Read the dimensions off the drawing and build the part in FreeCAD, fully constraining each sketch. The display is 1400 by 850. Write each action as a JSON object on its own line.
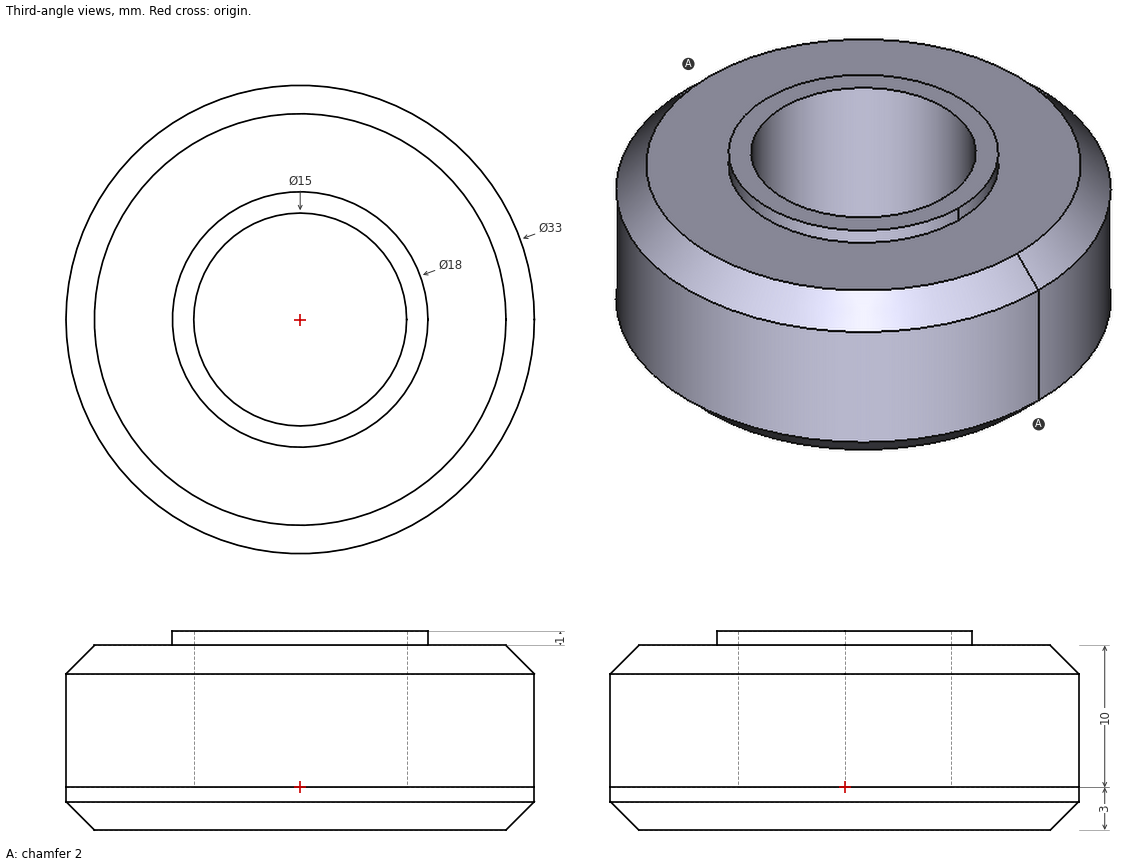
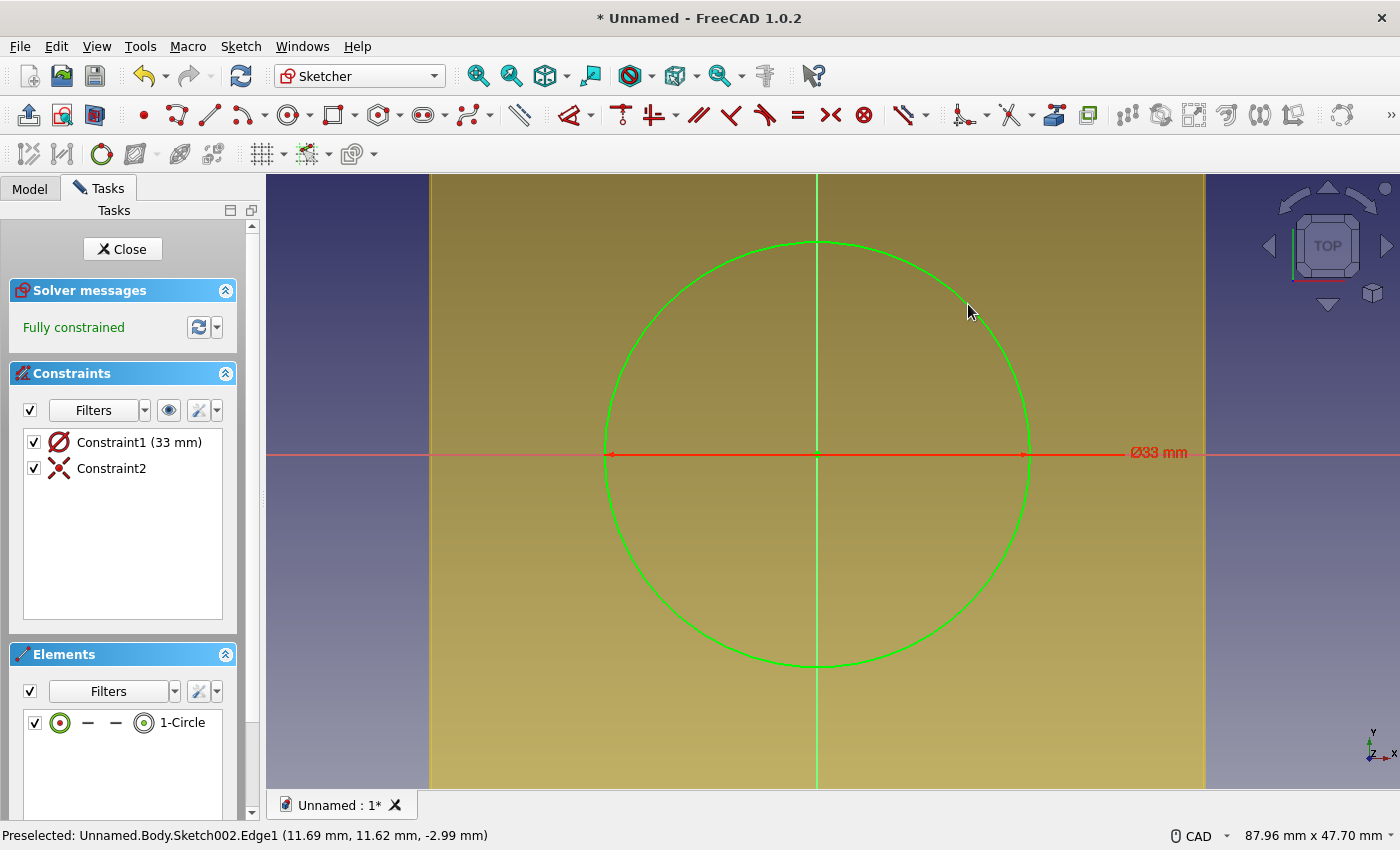
{"action": "left_click", "coordinate": [123, 249]}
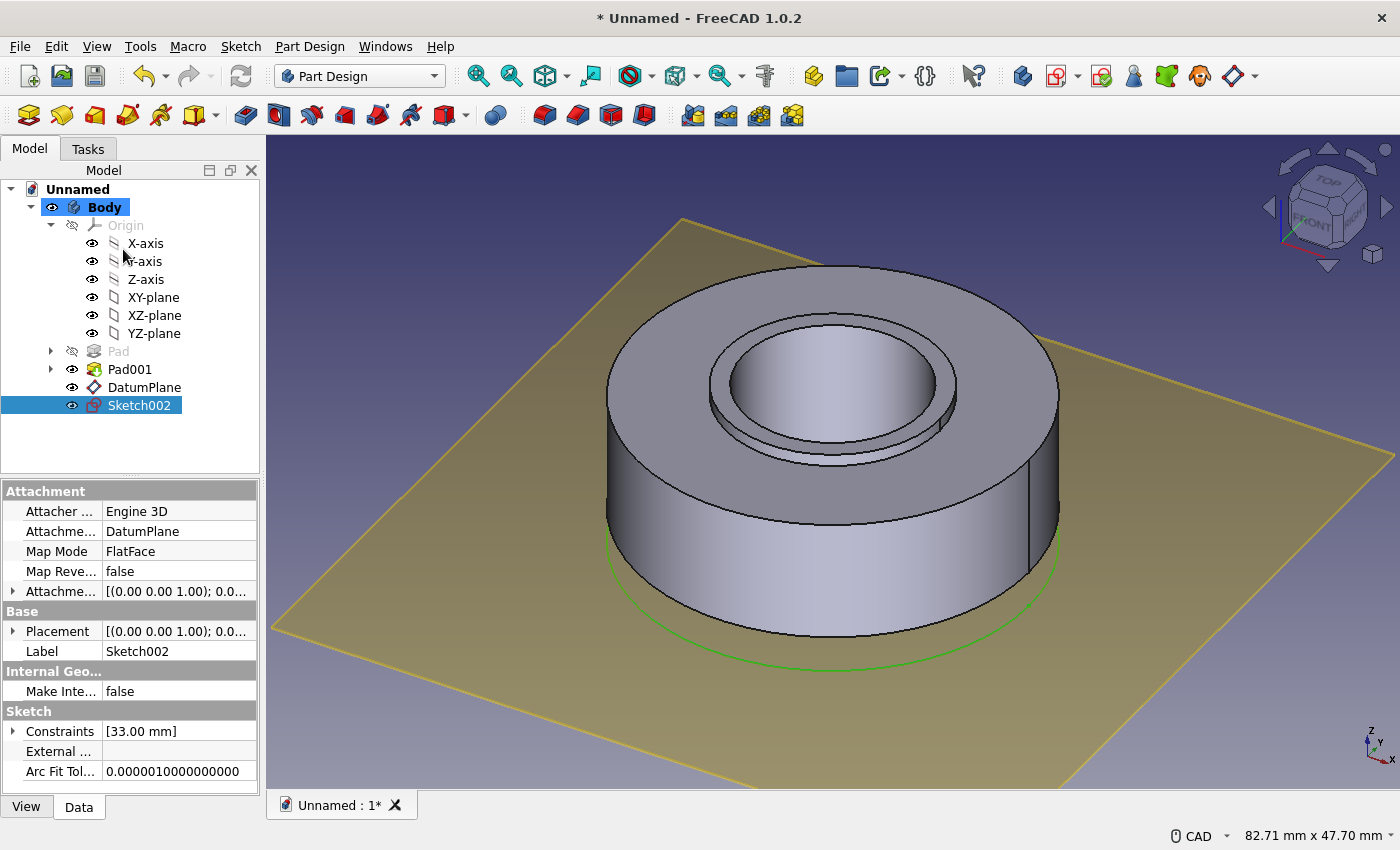
{"action": "left_click", "coordinate": [29, 116]}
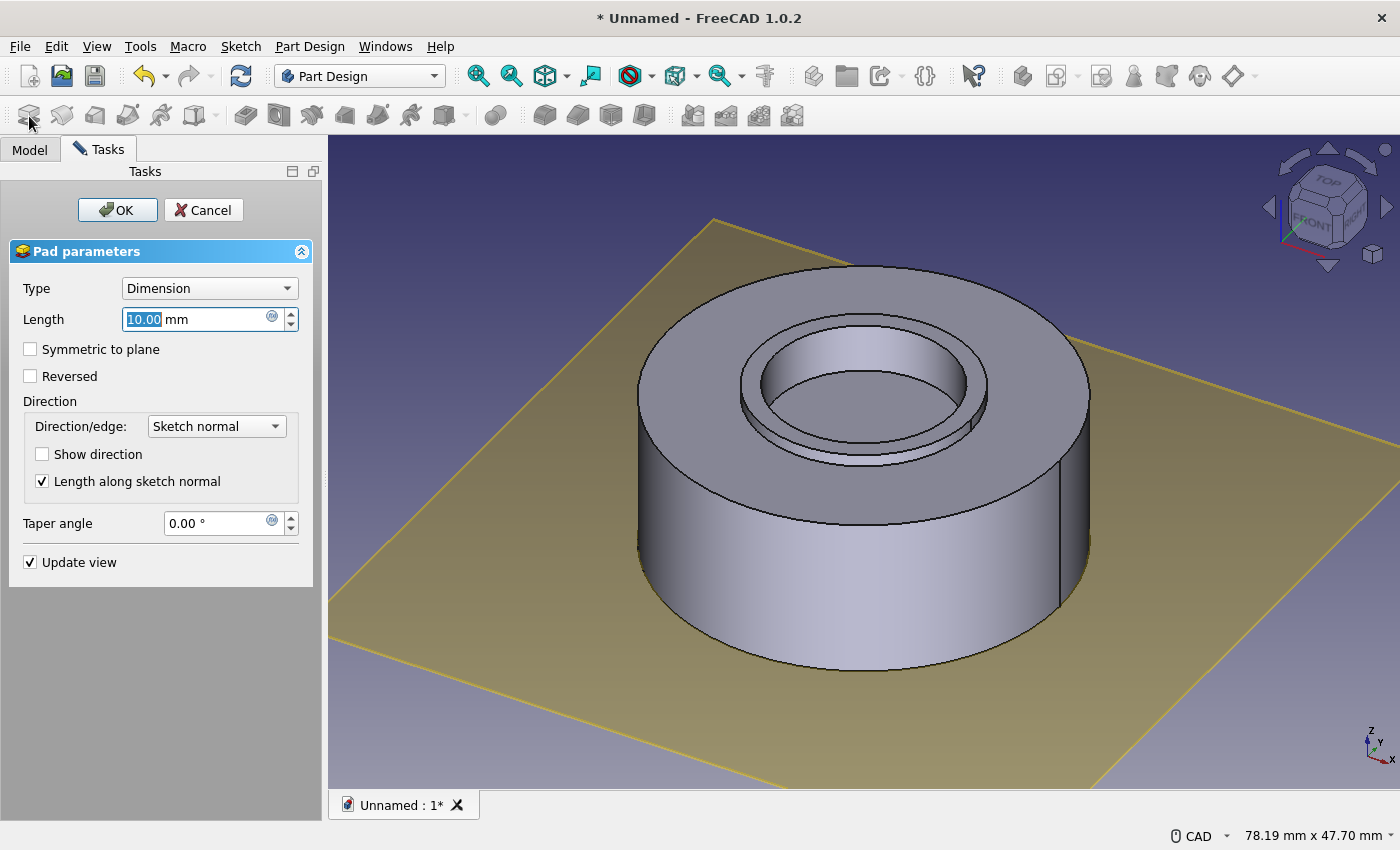
{"action": "type", "text": "3"}
{"action": "key", "text": "Tab"}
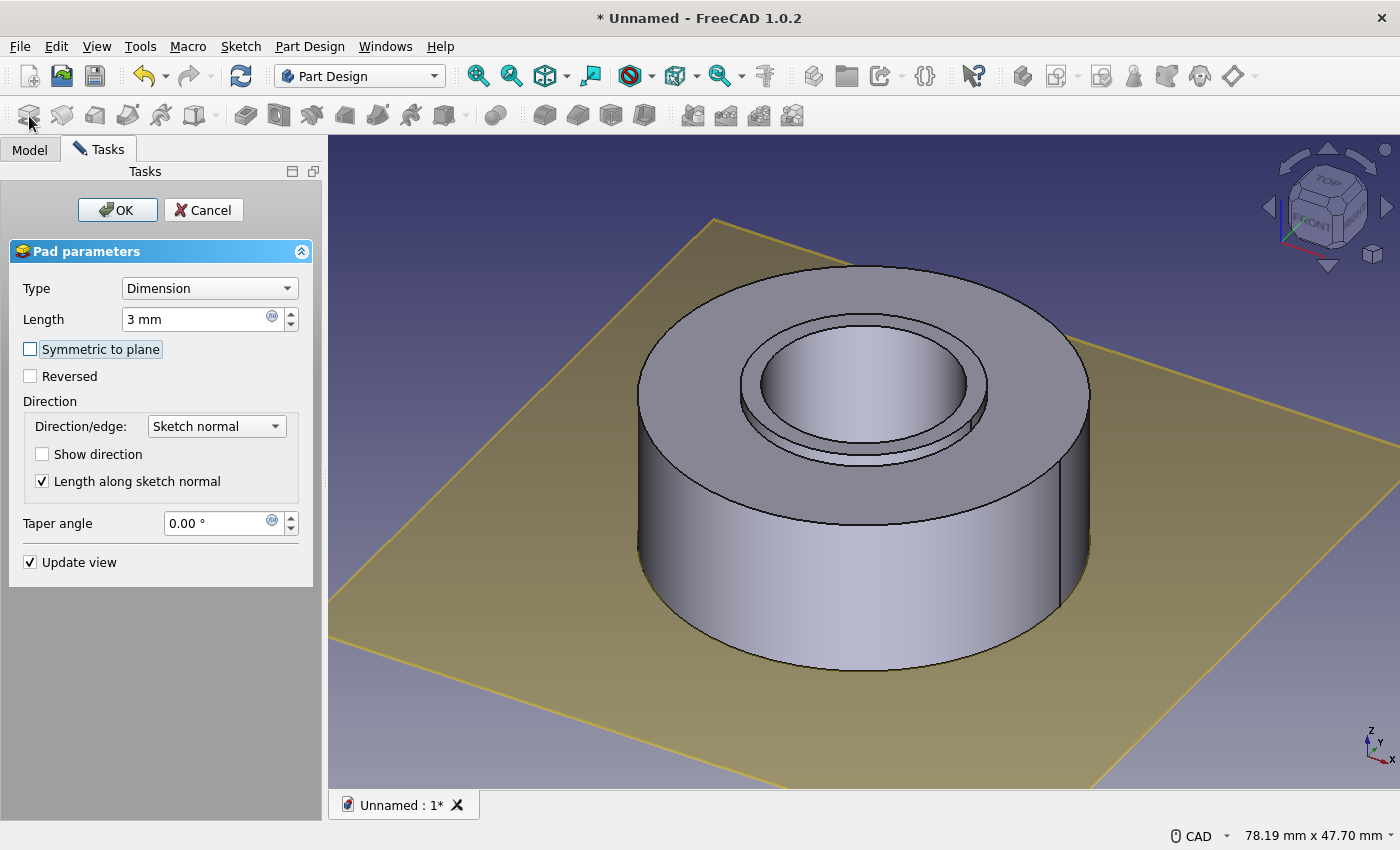
{"action": "left_click", "coordinate": [118, 210]}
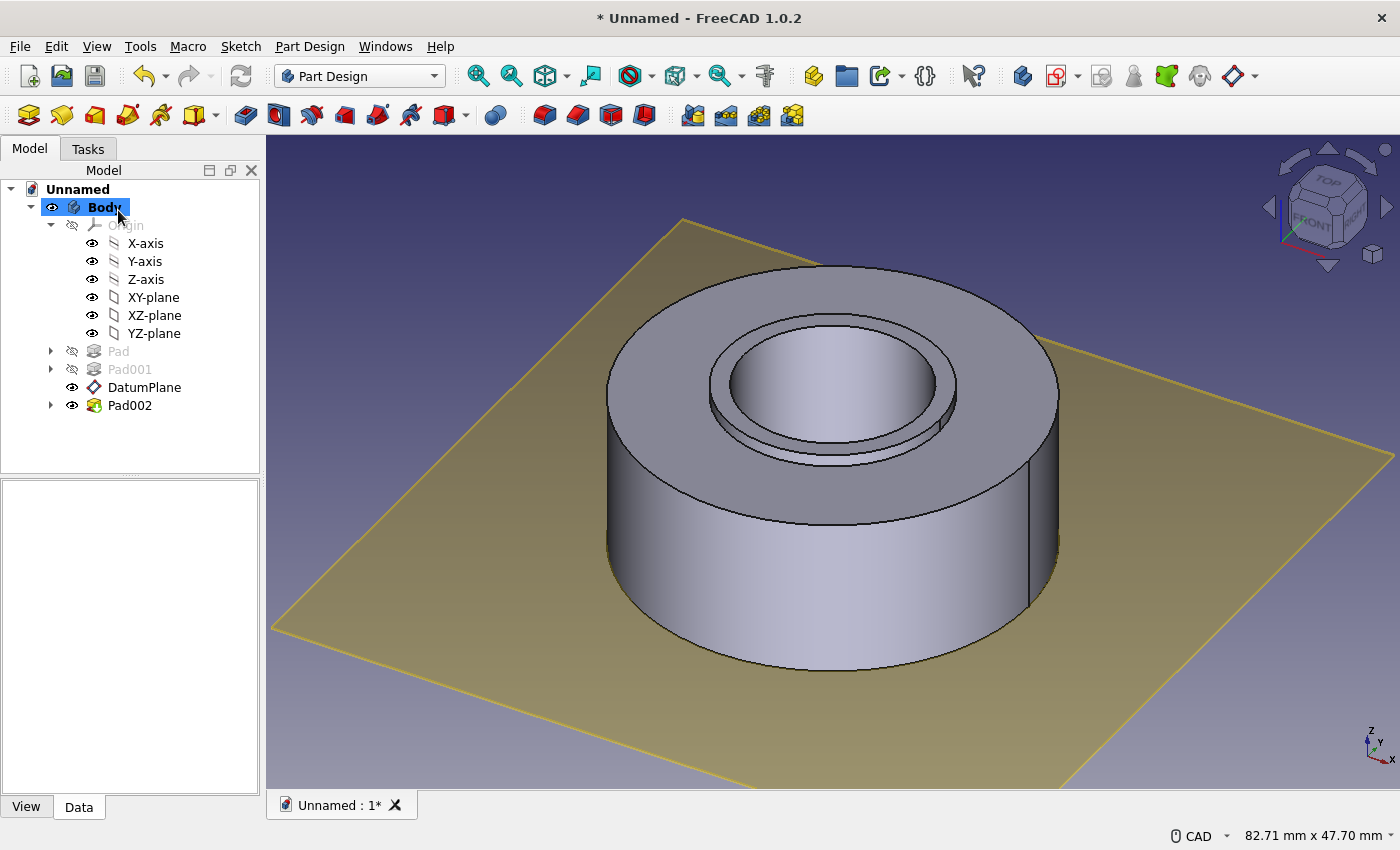
{"action": "left_click", "coordinate": [117, 387]}
{"action": "key", "text": "space"}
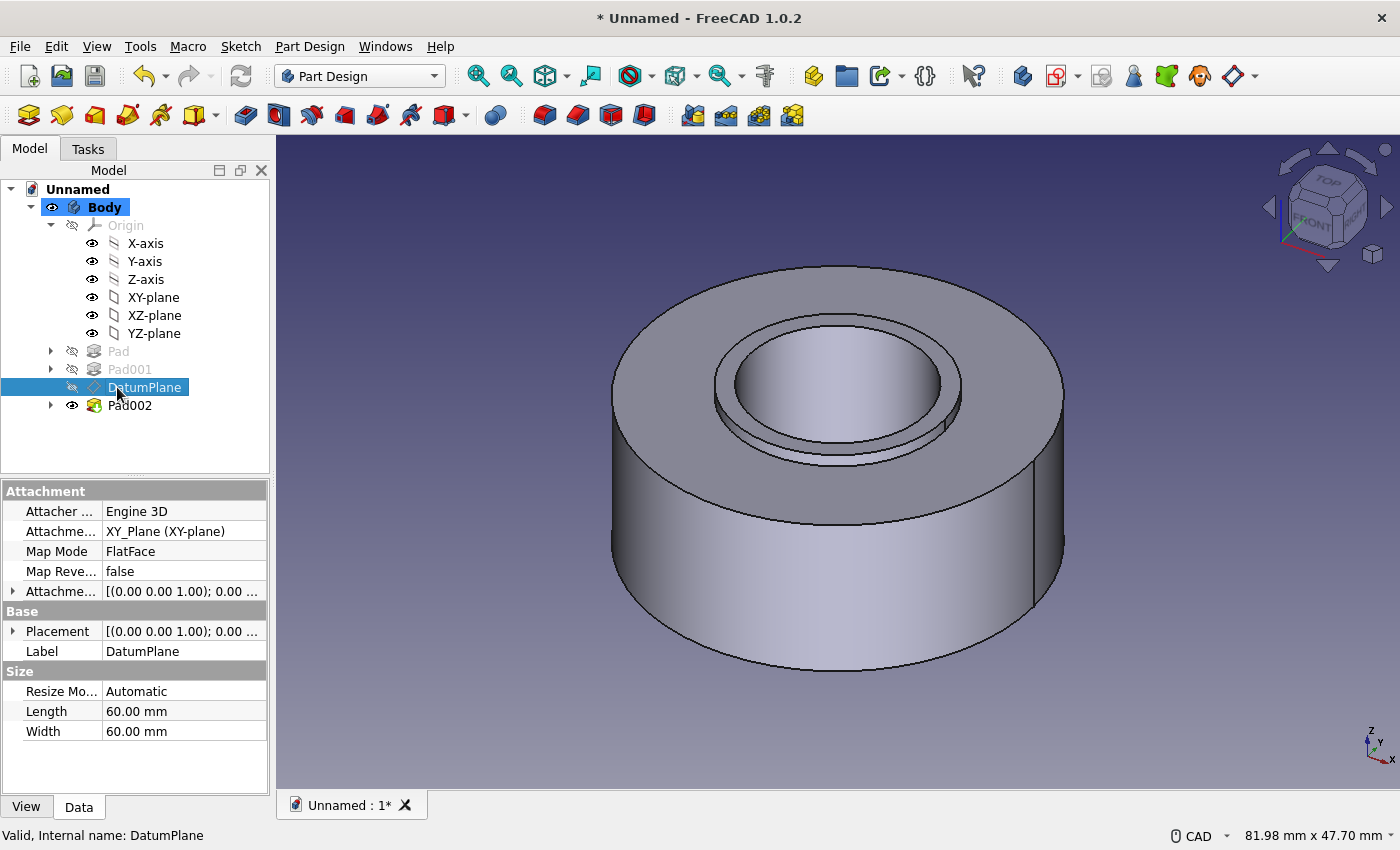
{"action": "left_click", "coordinate": [613, 408]}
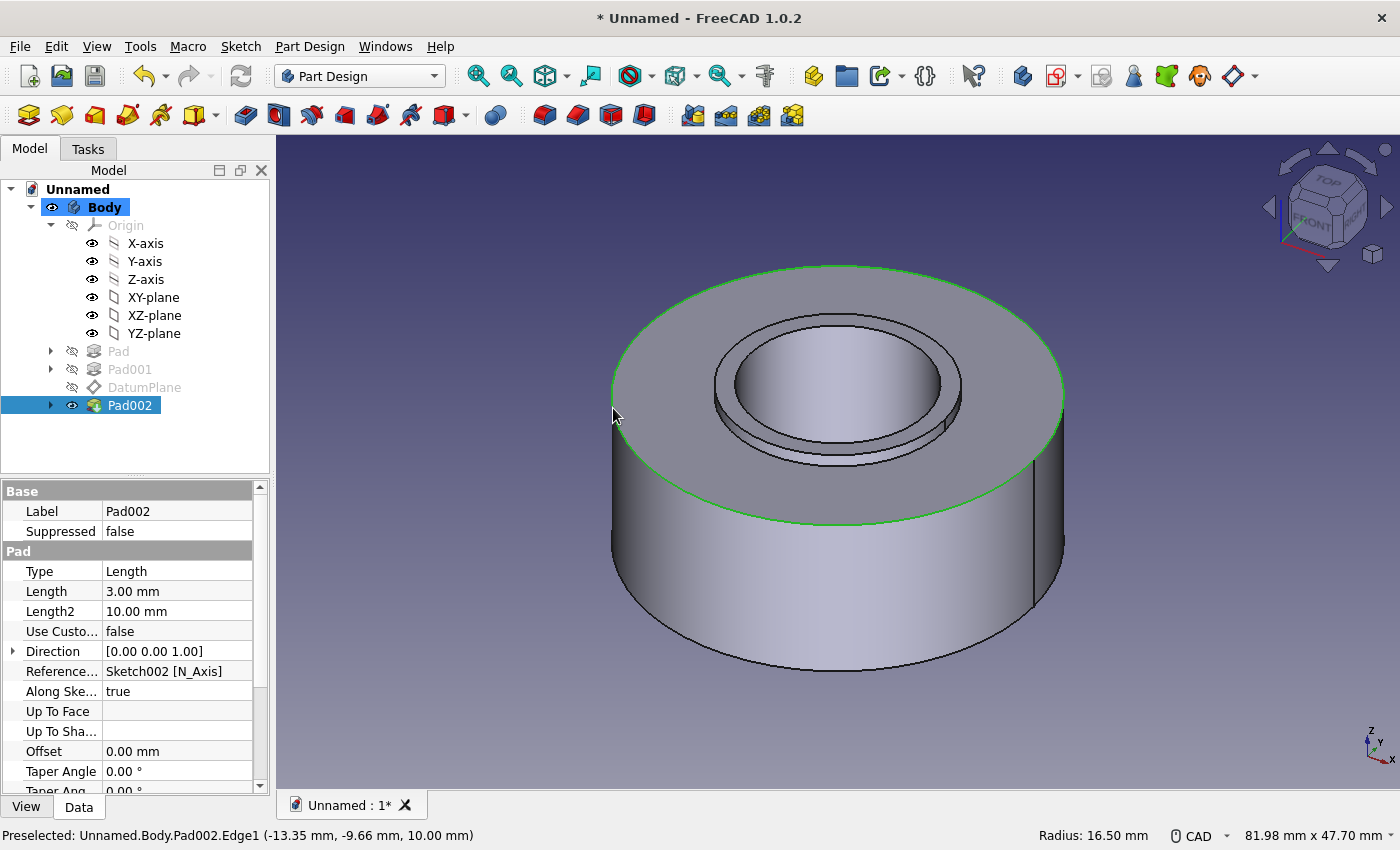
{"action": "key", "text": "0"}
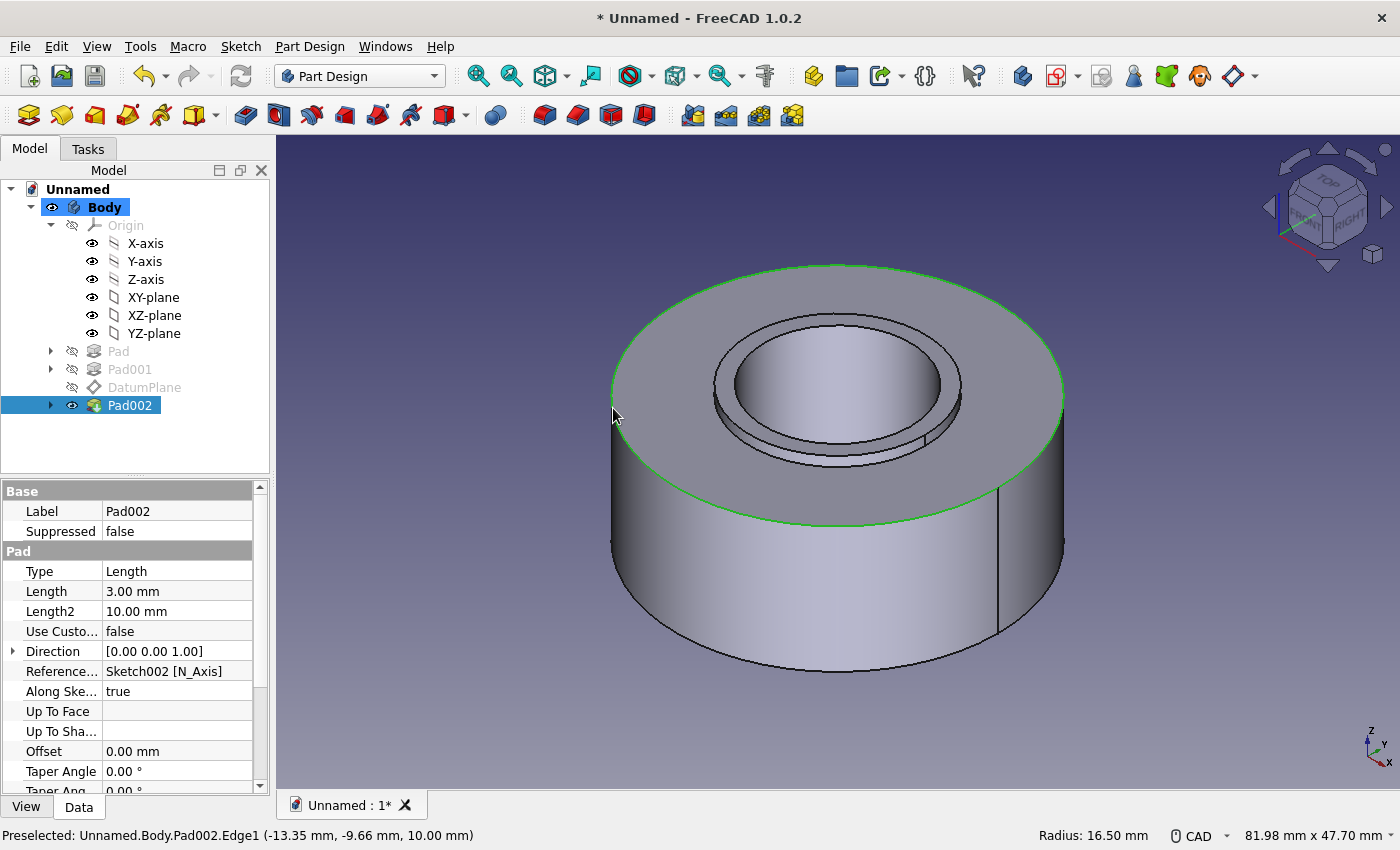
{"action": "key", "text": "2"}